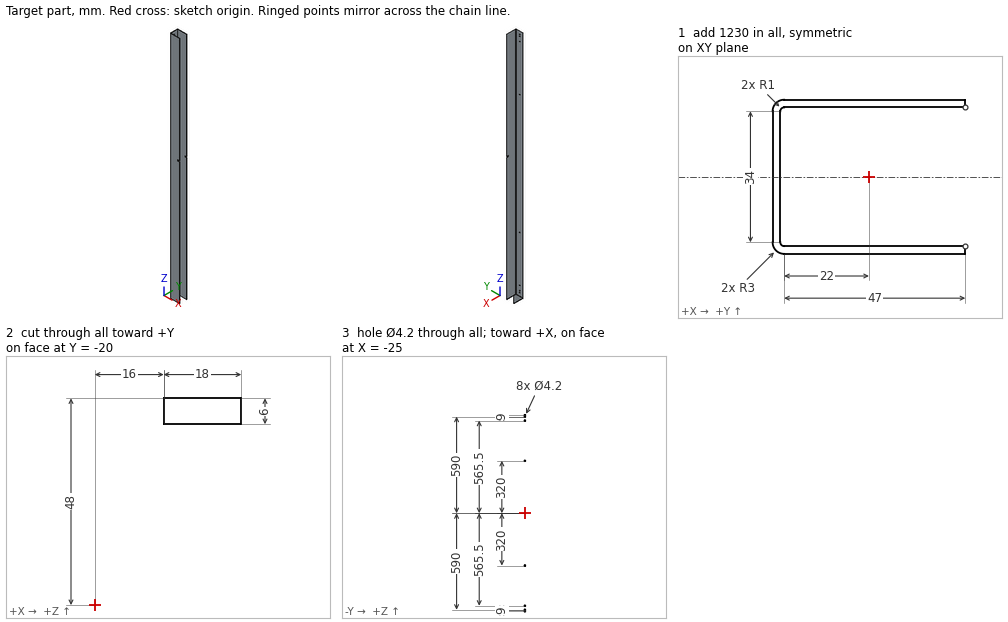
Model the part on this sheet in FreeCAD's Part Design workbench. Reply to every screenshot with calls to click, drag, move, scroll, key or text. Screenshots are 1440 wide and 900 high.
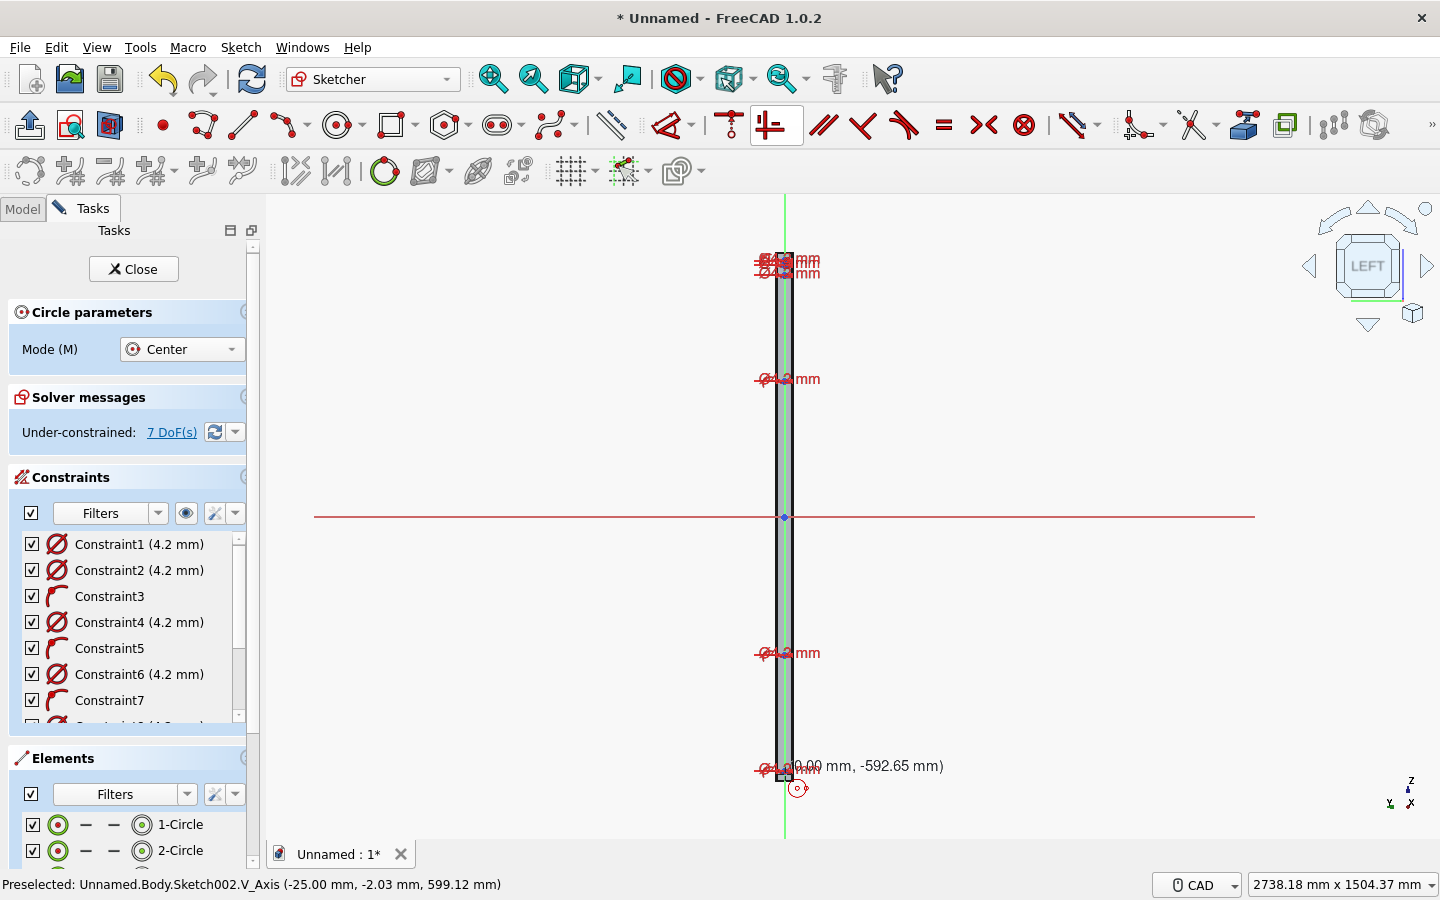
scroll(785, 774, up, 9)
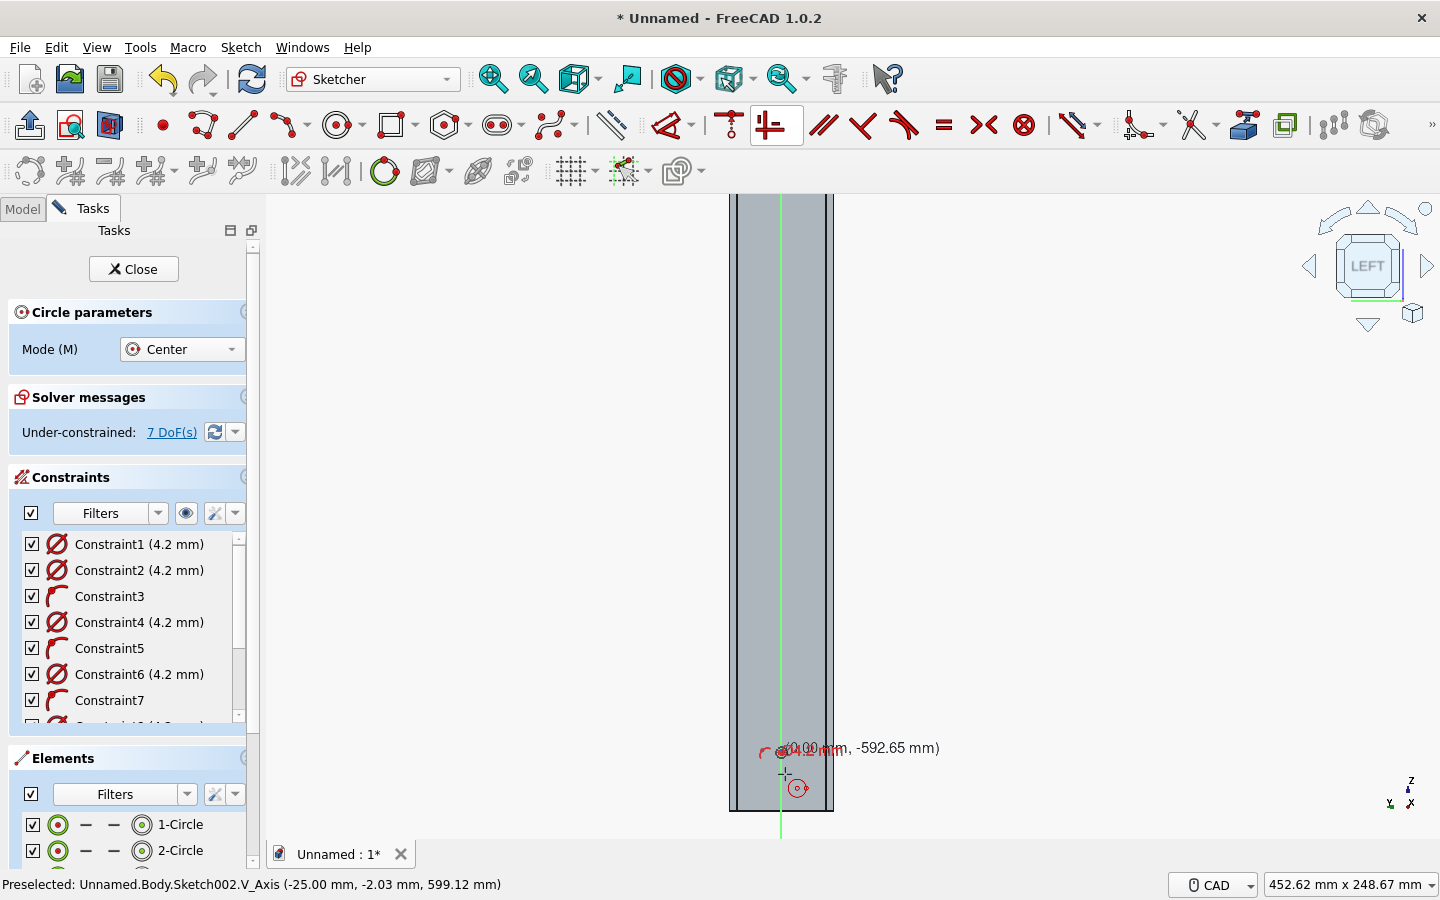
click(781, 769)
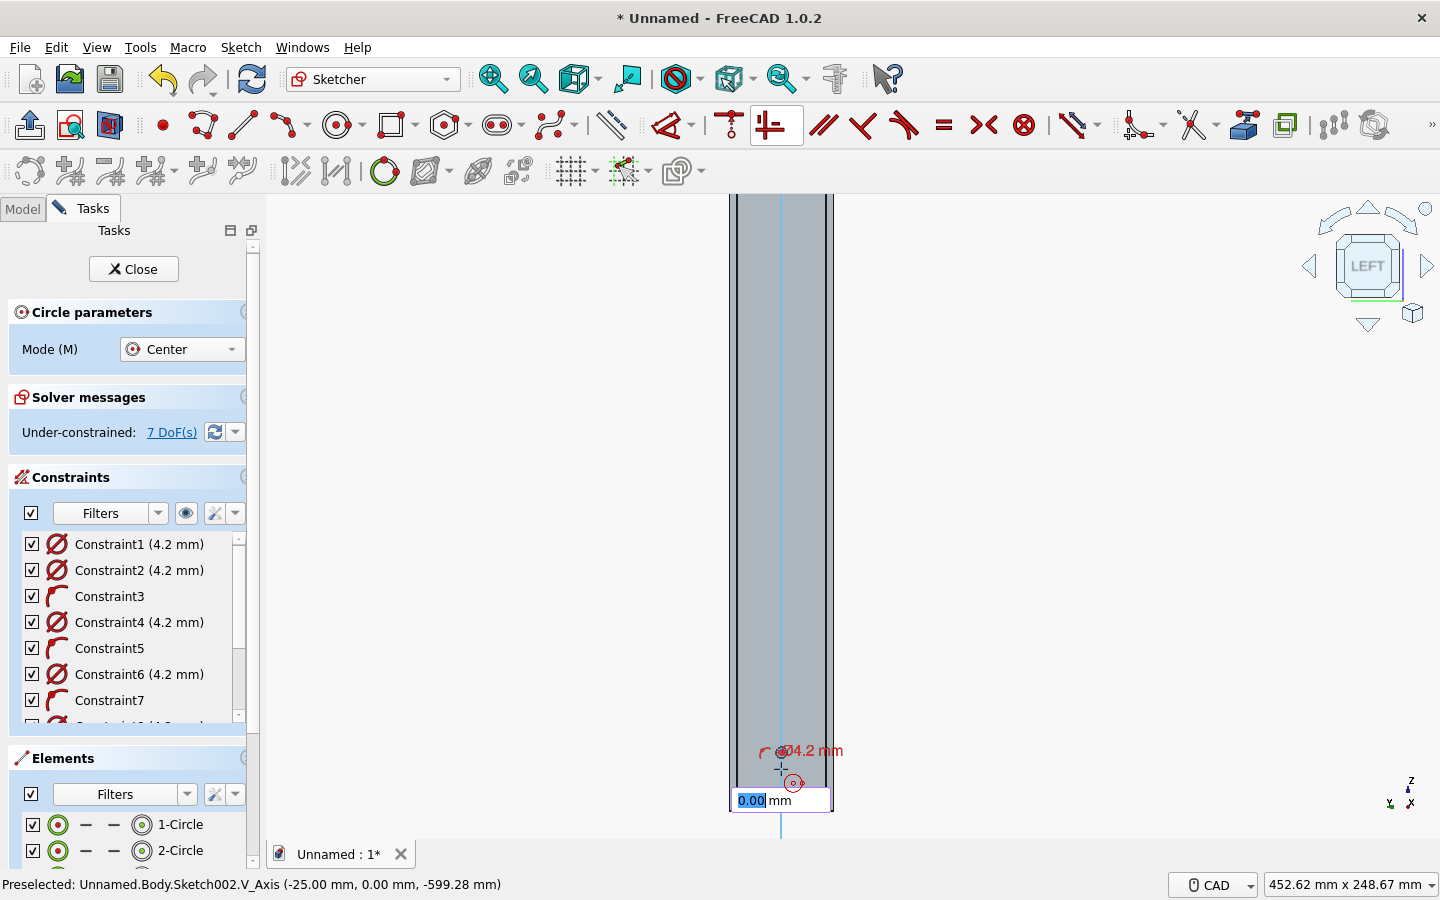
scroll(787, 767, up, 6)
move(785, 766)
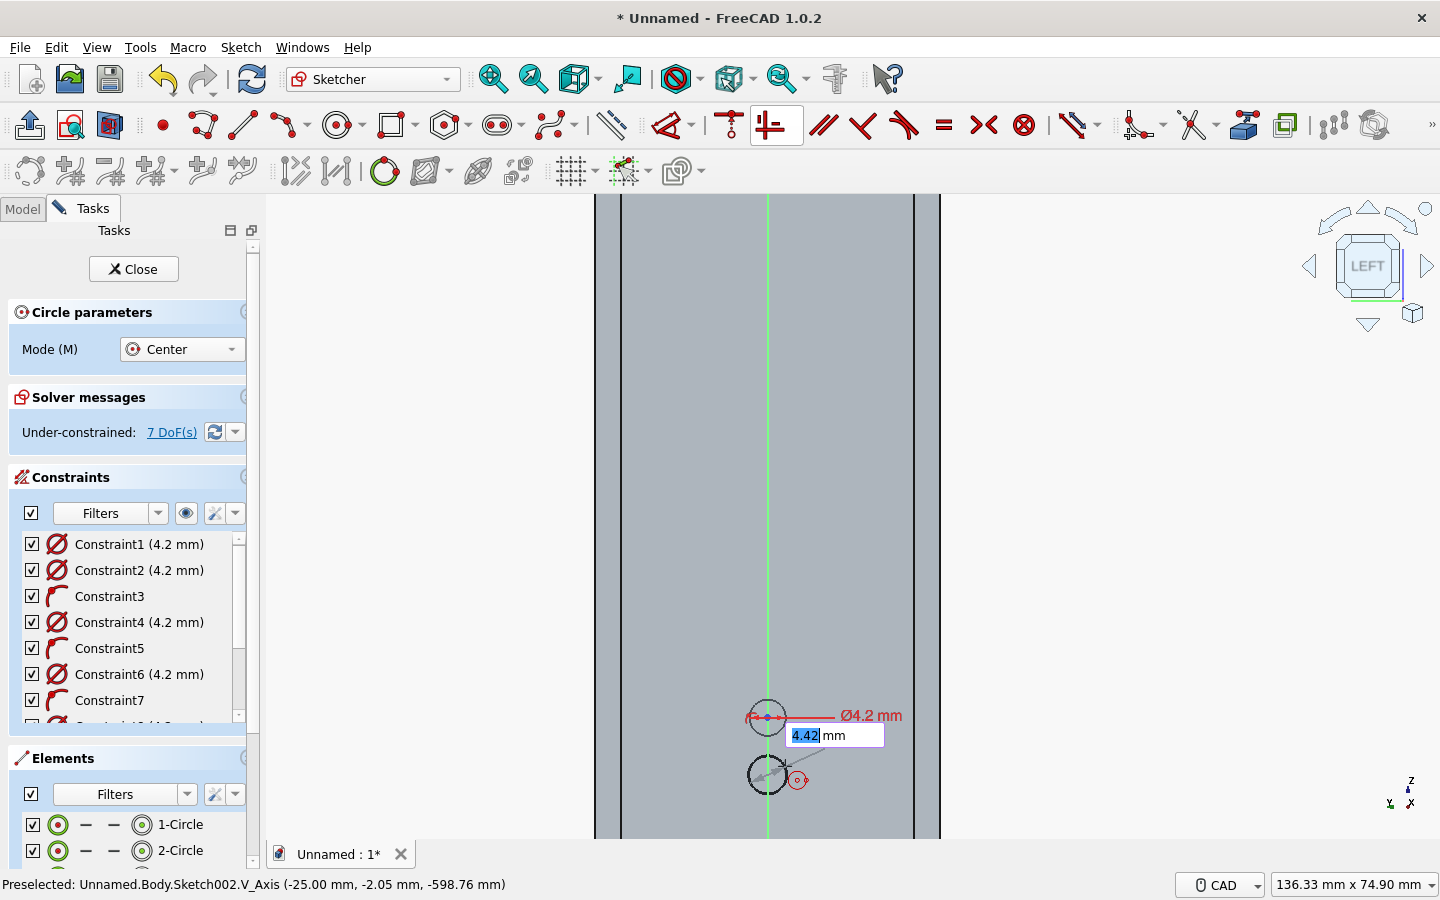
text(4.2)
key(Return)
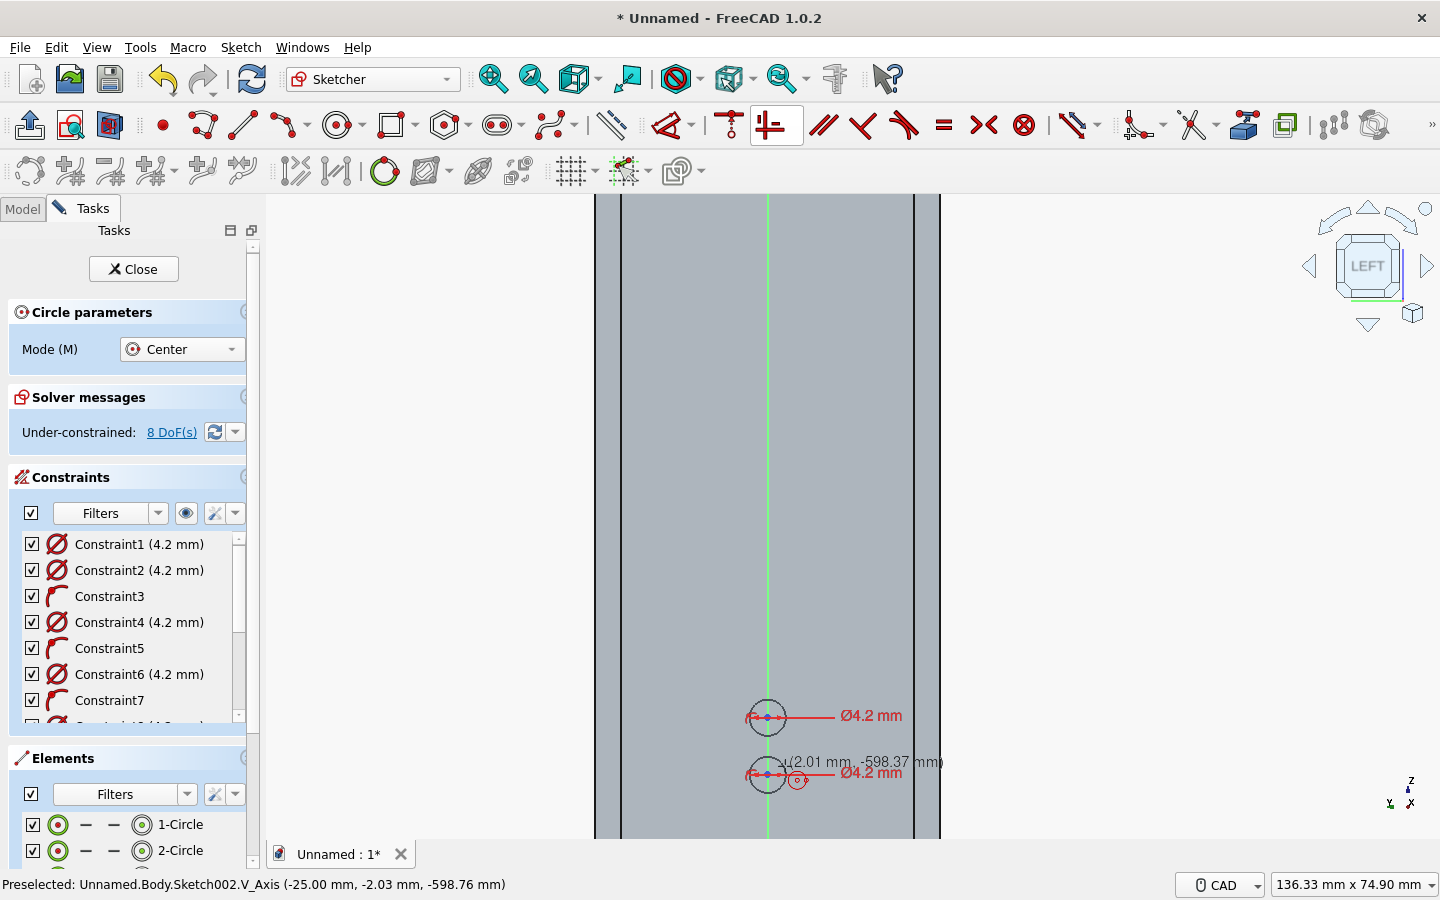
scroll(768, 484, up, 2)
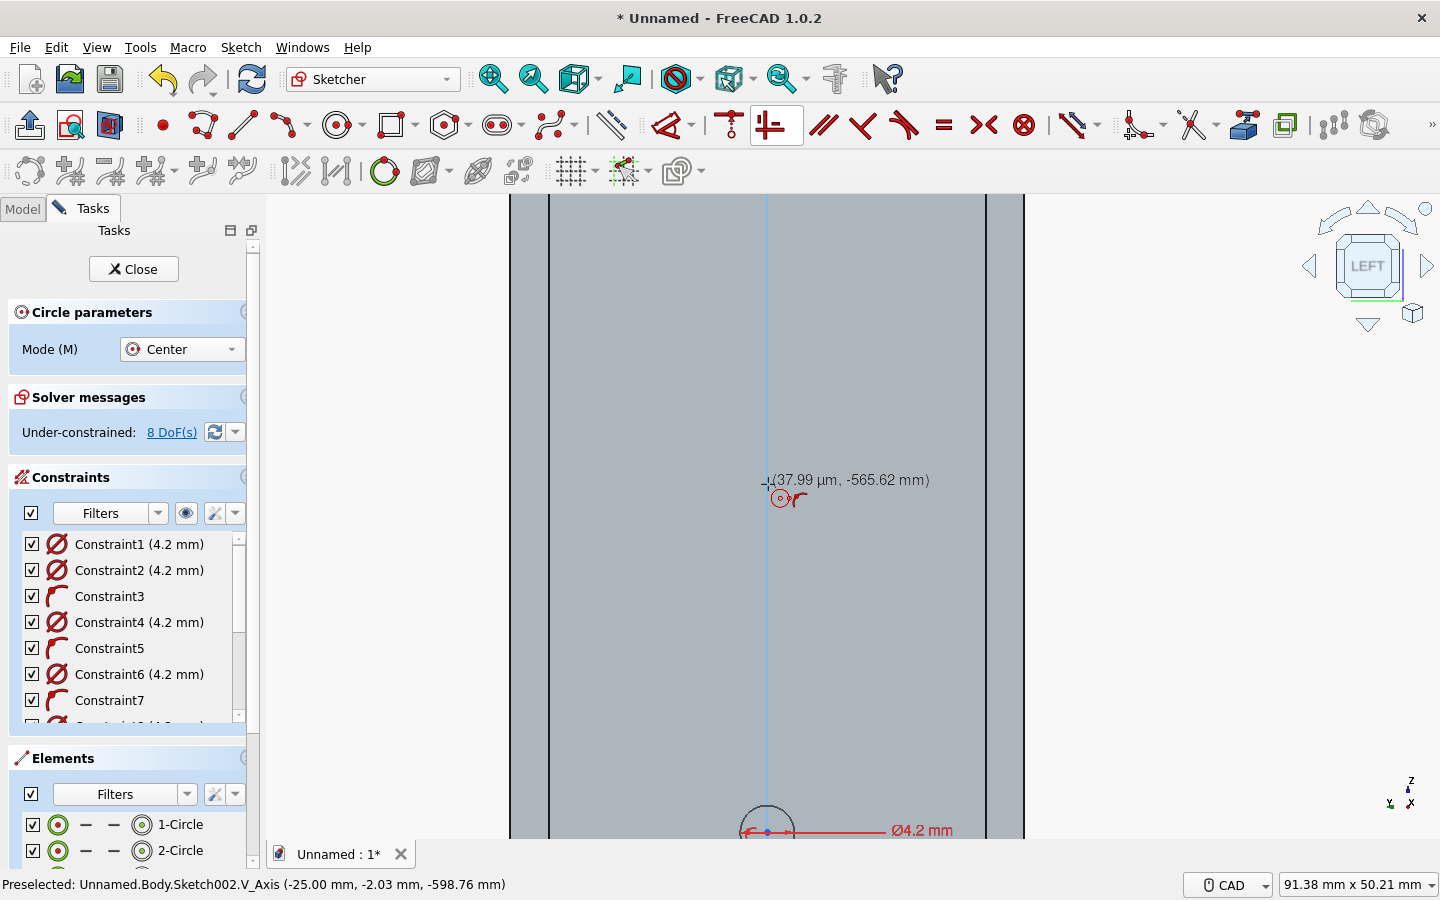
scroll(785, 768, down, 17)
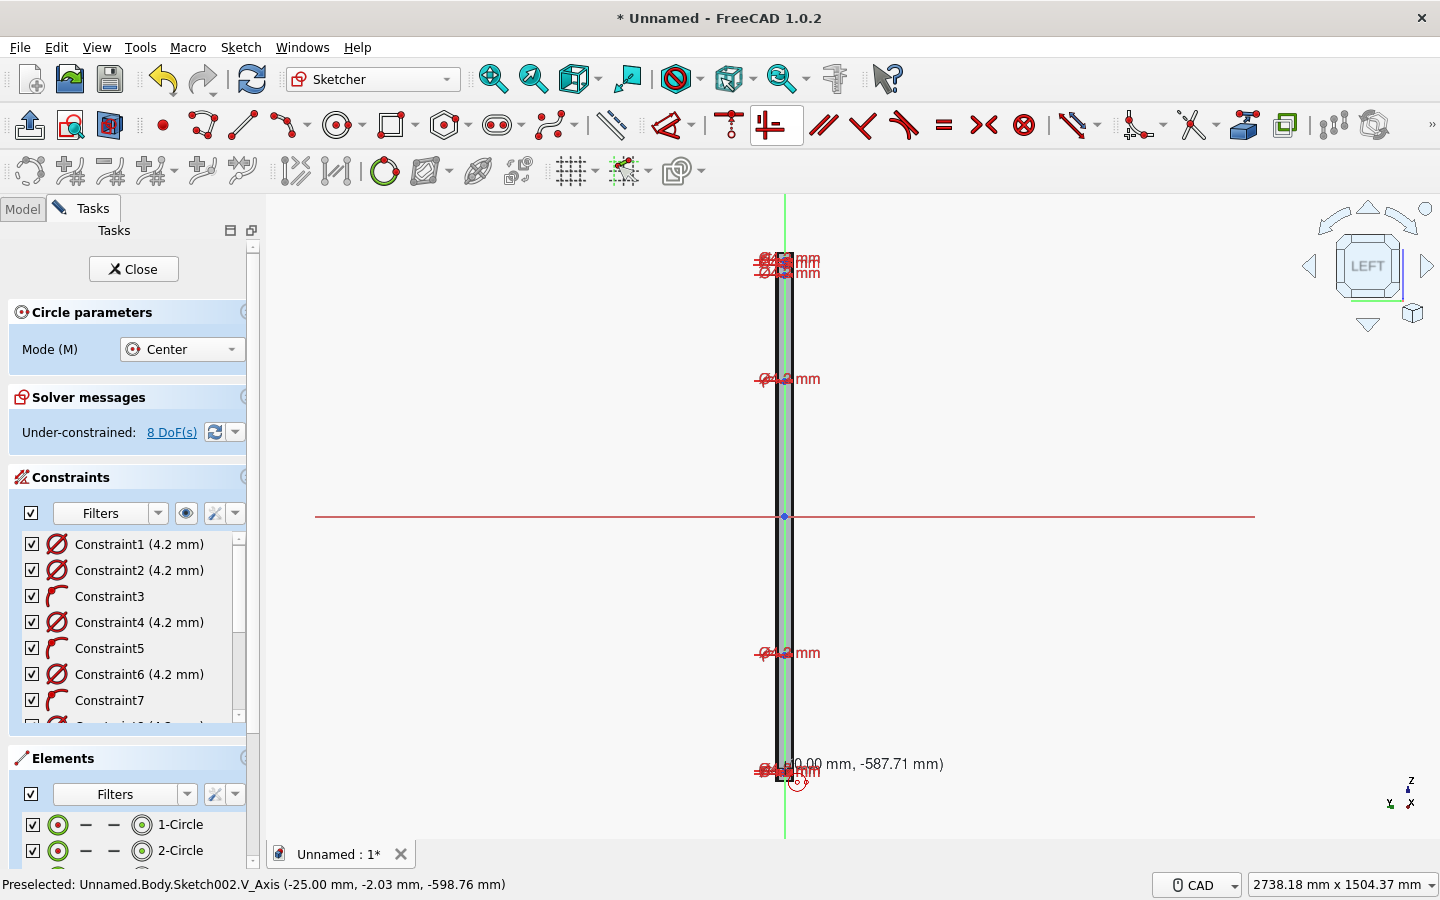
scroll(785, 759, up, 3)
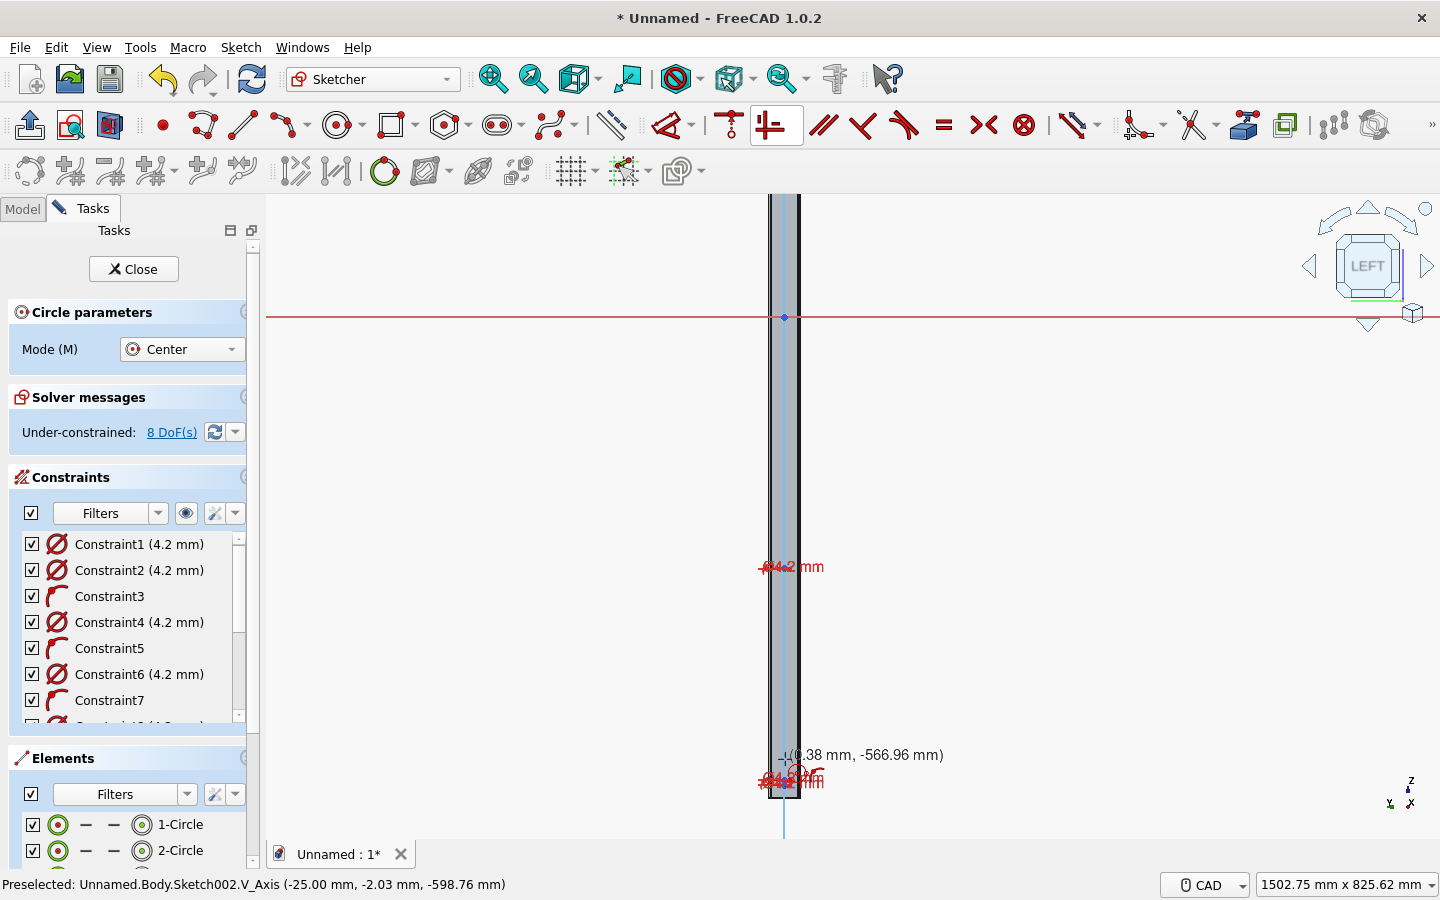
click(784, 759)